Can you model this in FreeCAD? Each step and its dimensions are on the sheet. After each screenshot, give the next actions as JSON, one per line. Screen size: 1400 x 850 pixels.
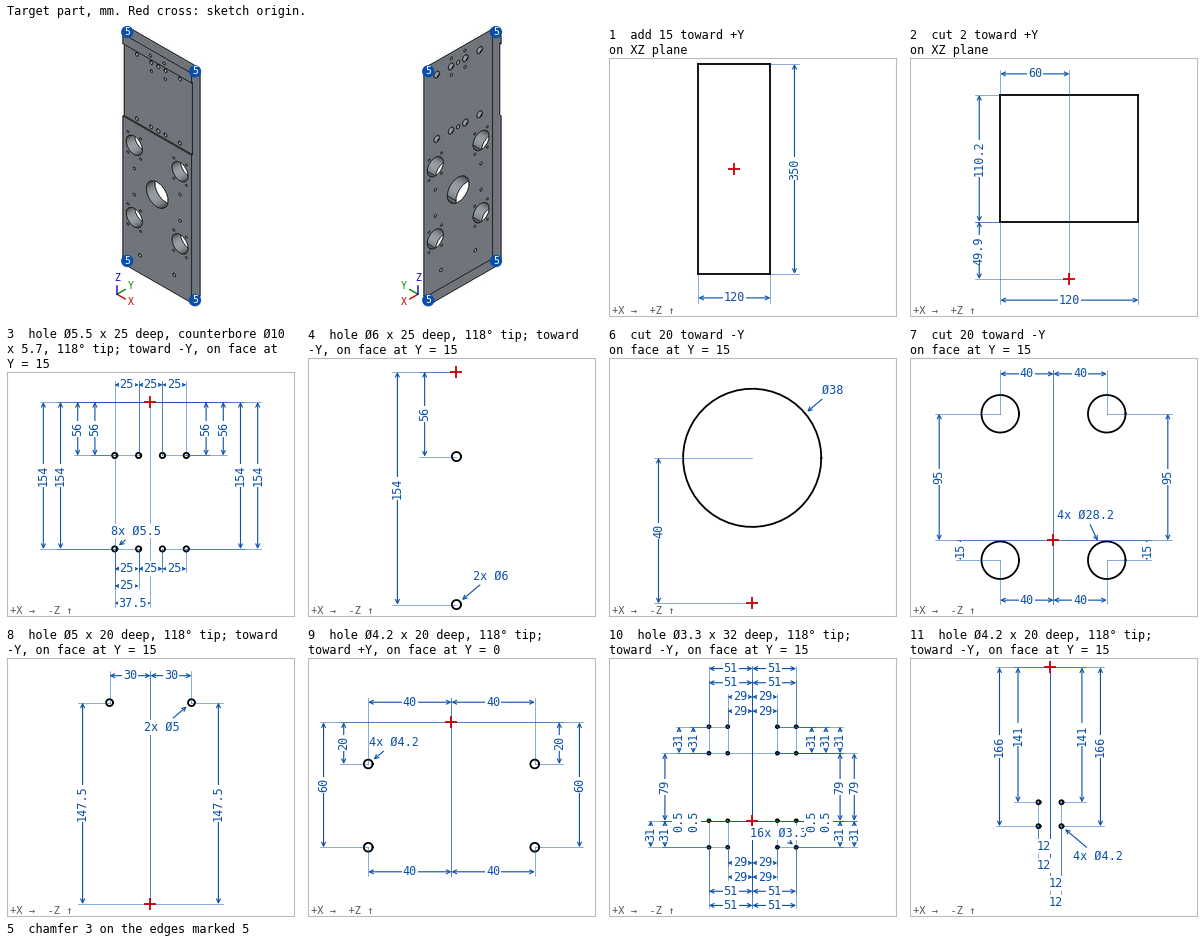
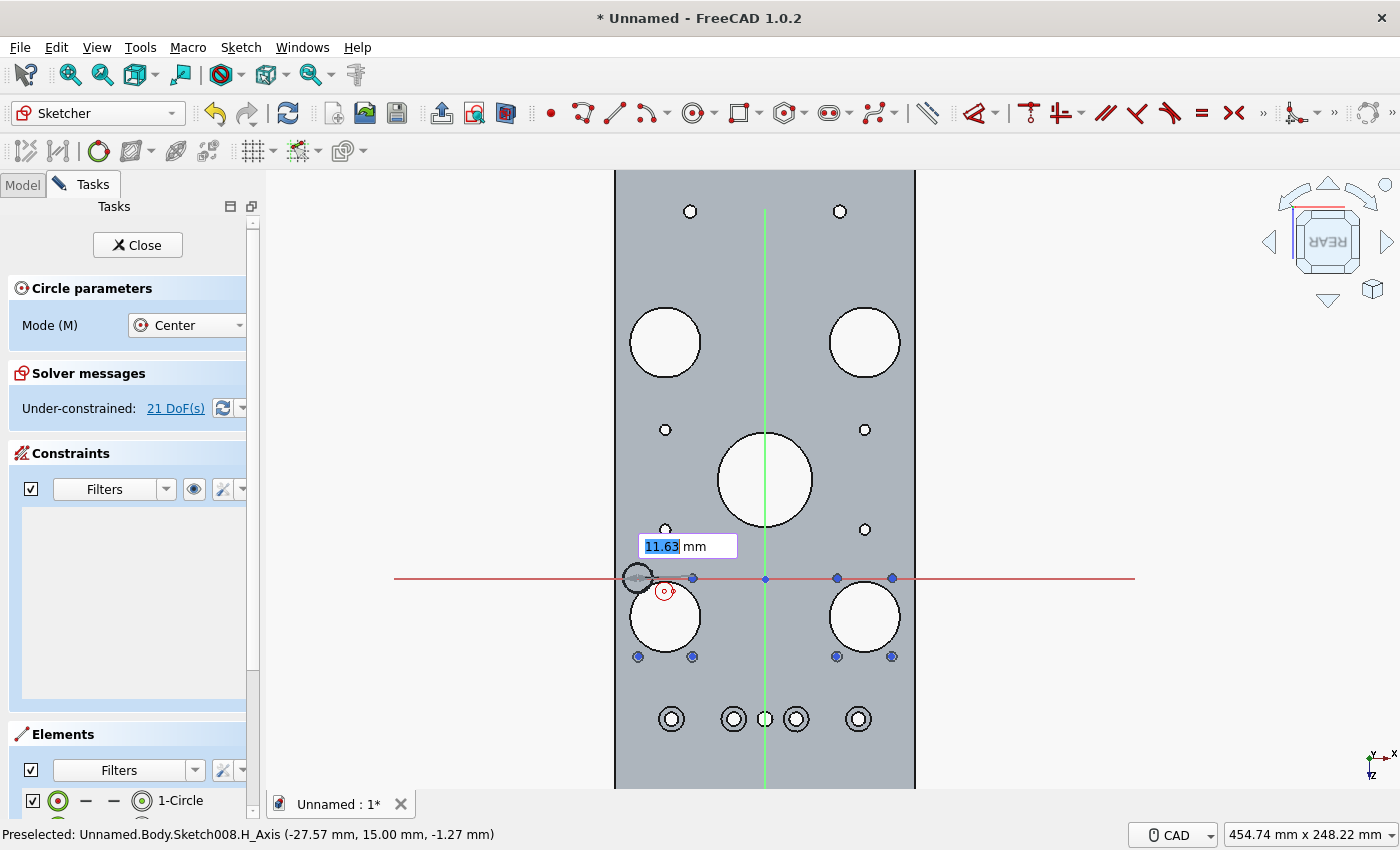
{"action": "scroll", "coordinate": [641, 575], "scroll_direction": "up", "scroll_amount": 7}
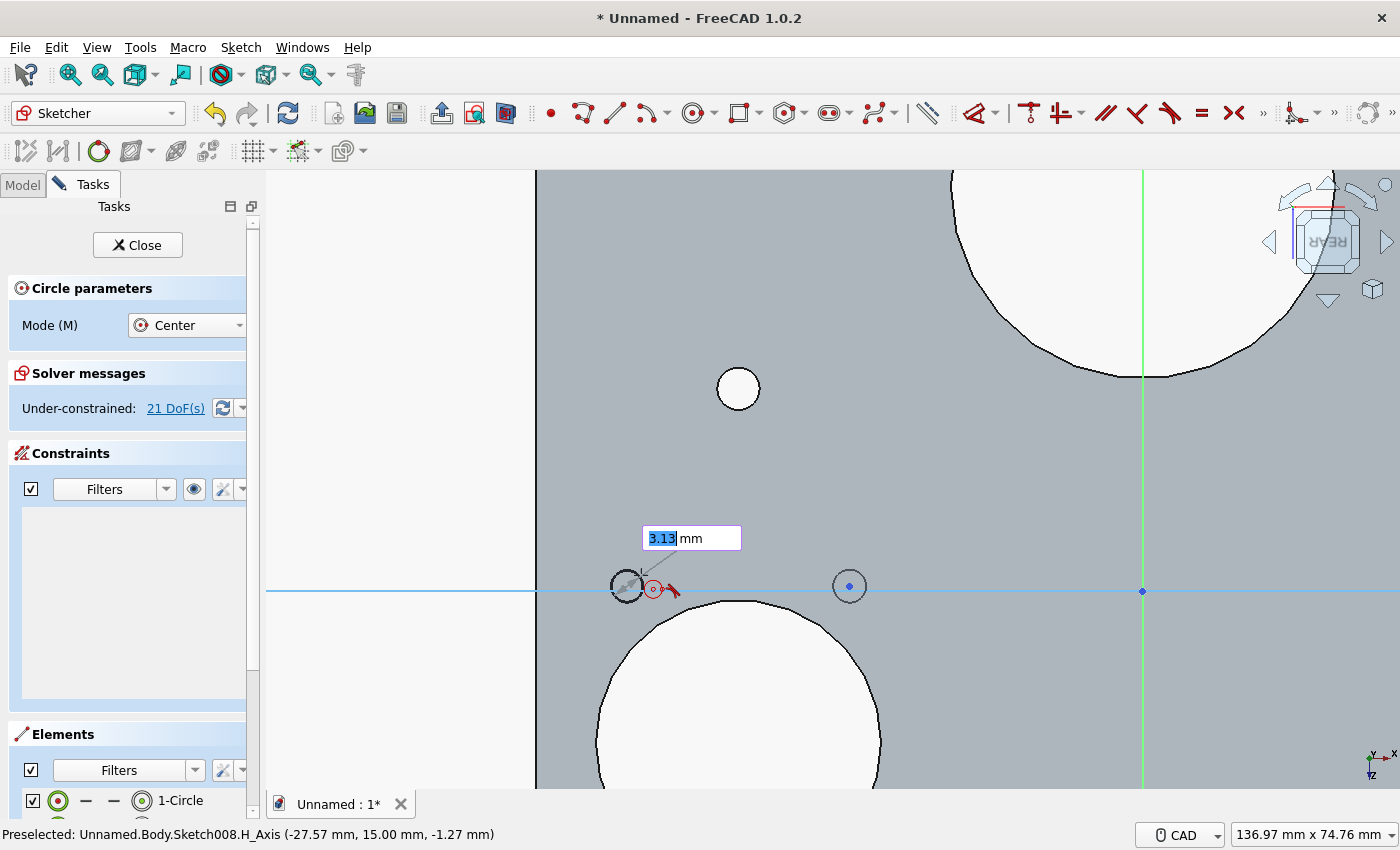
{"action": "left_click", "coordinate": [639, 574]}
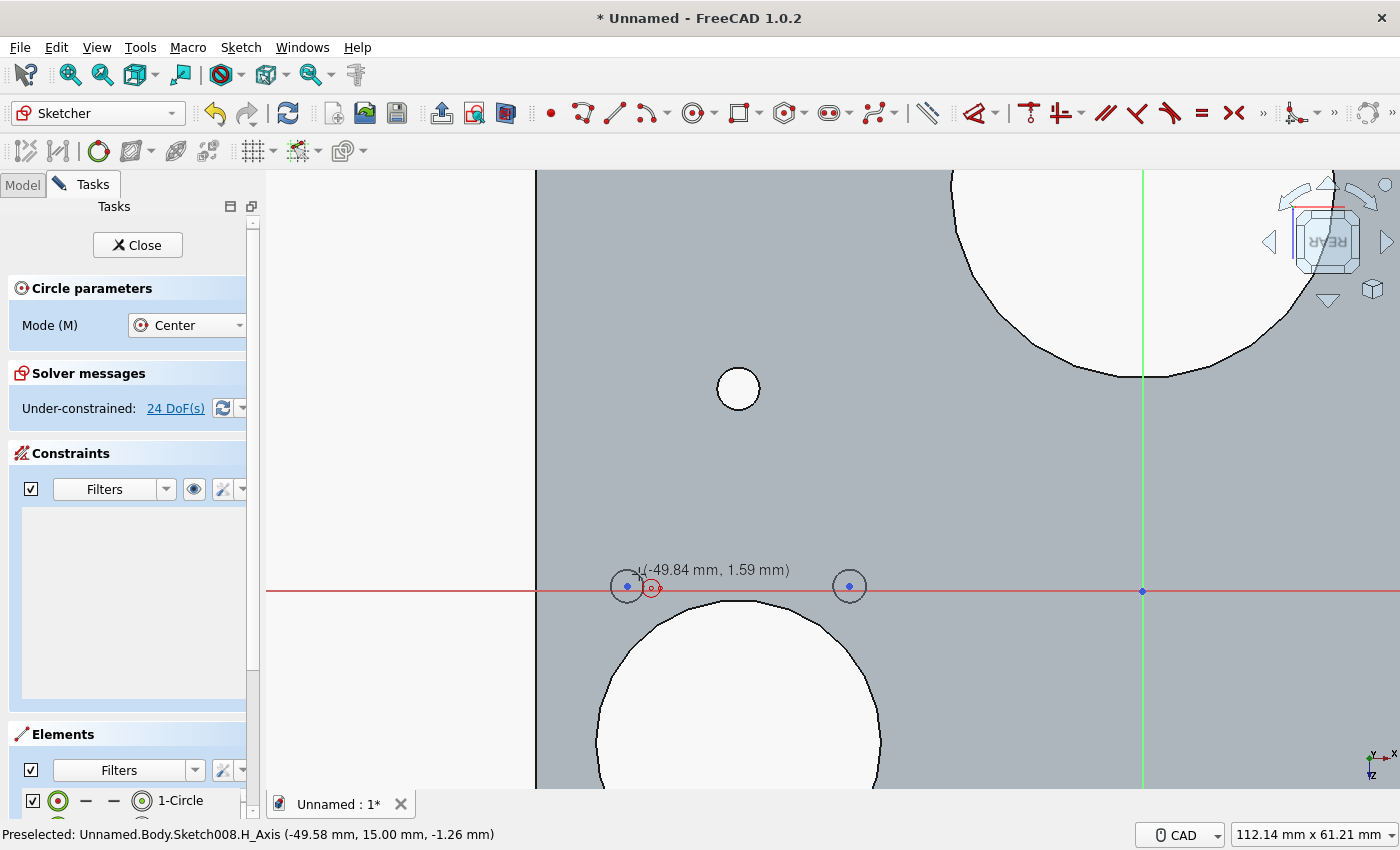
{"action": "scroll", "coordinate": [641, 575], "scroll_direction": "down", "scroll_amount": 7}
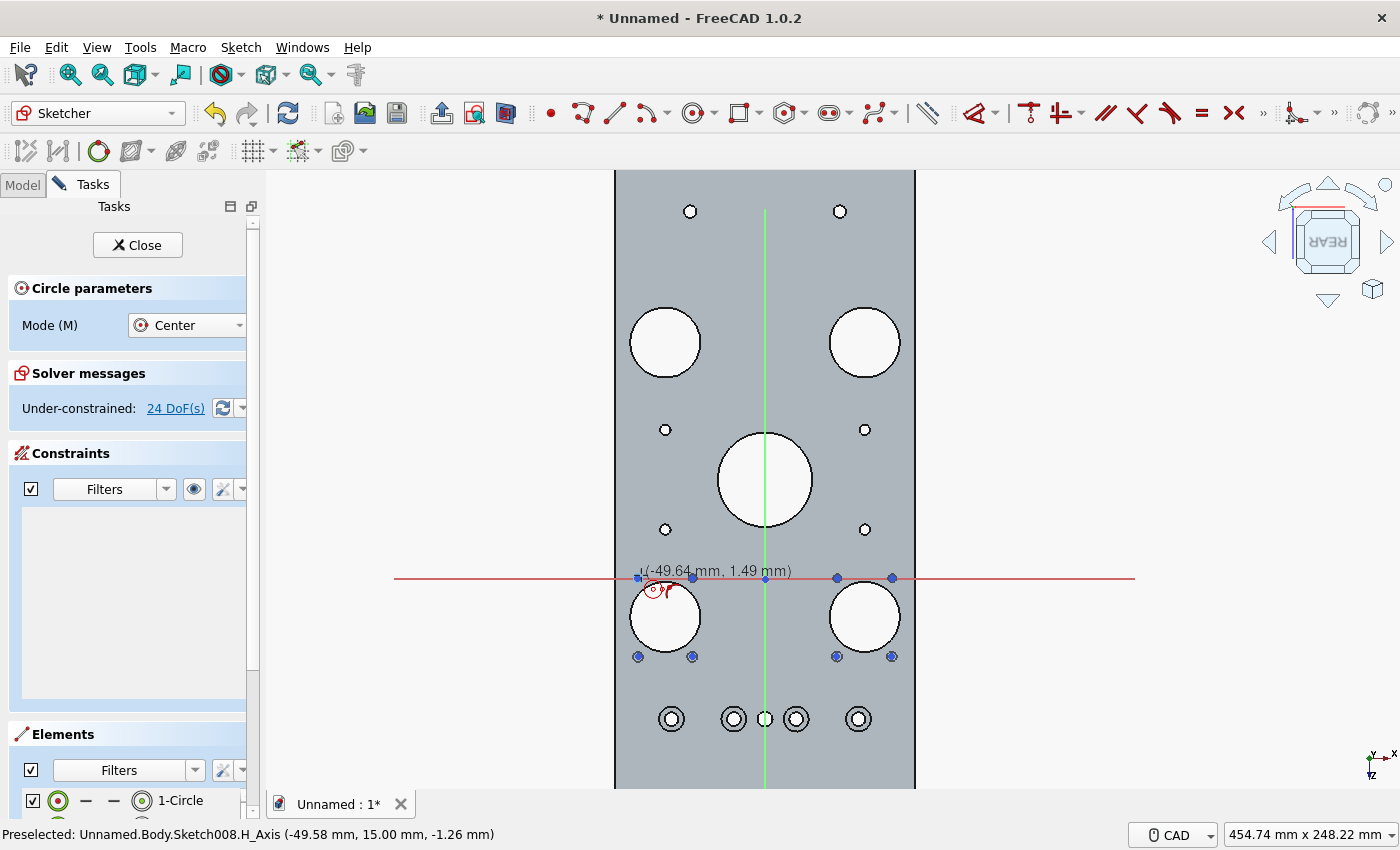
{"action": "scroll", "coordinate": [892, 381], "scroll_direction": "up", "scroll_amount": 9}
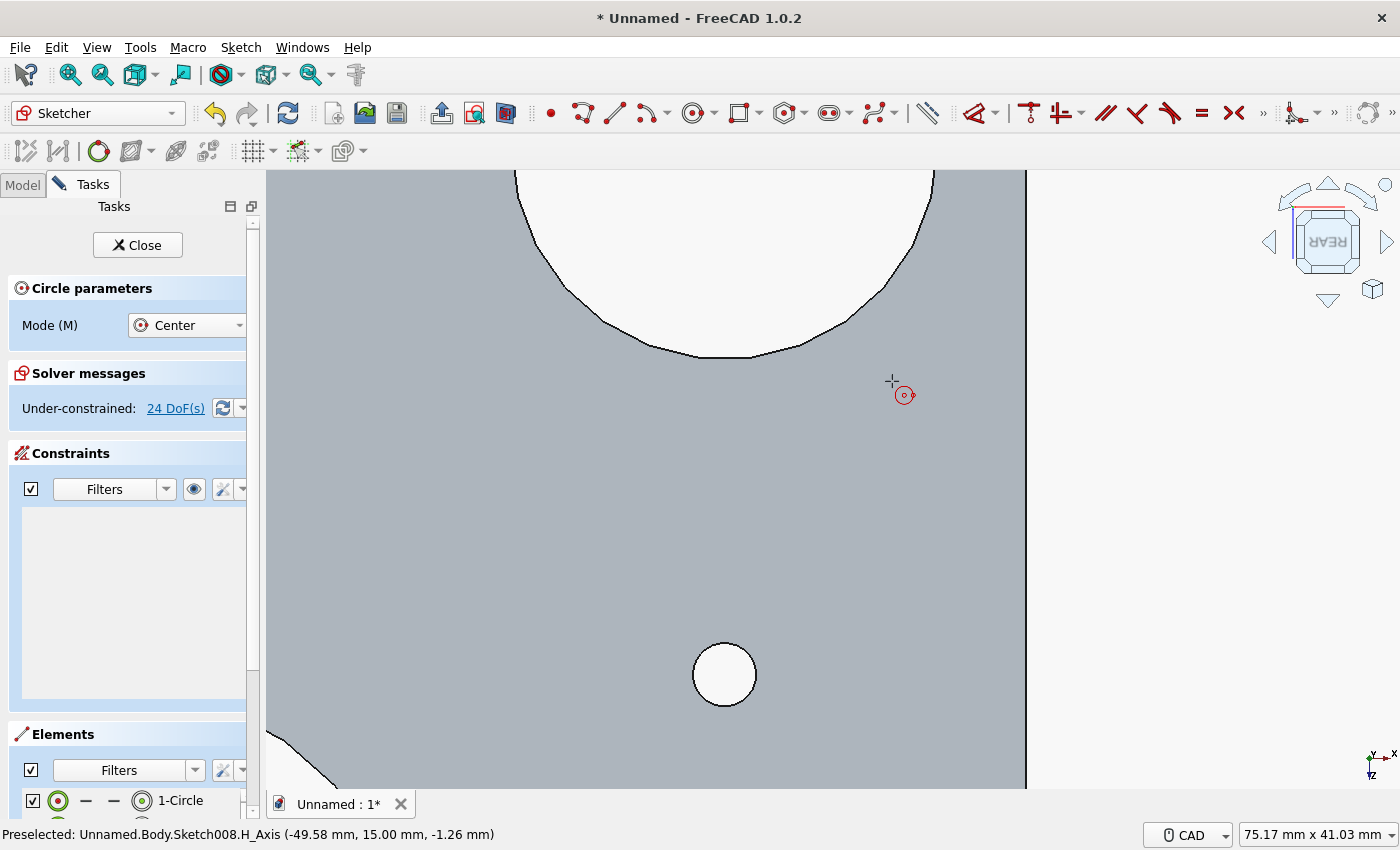
{"action": "scroll", "coordinate": [892, 381], "scroll_direction": "down", "scroll_amount": 9}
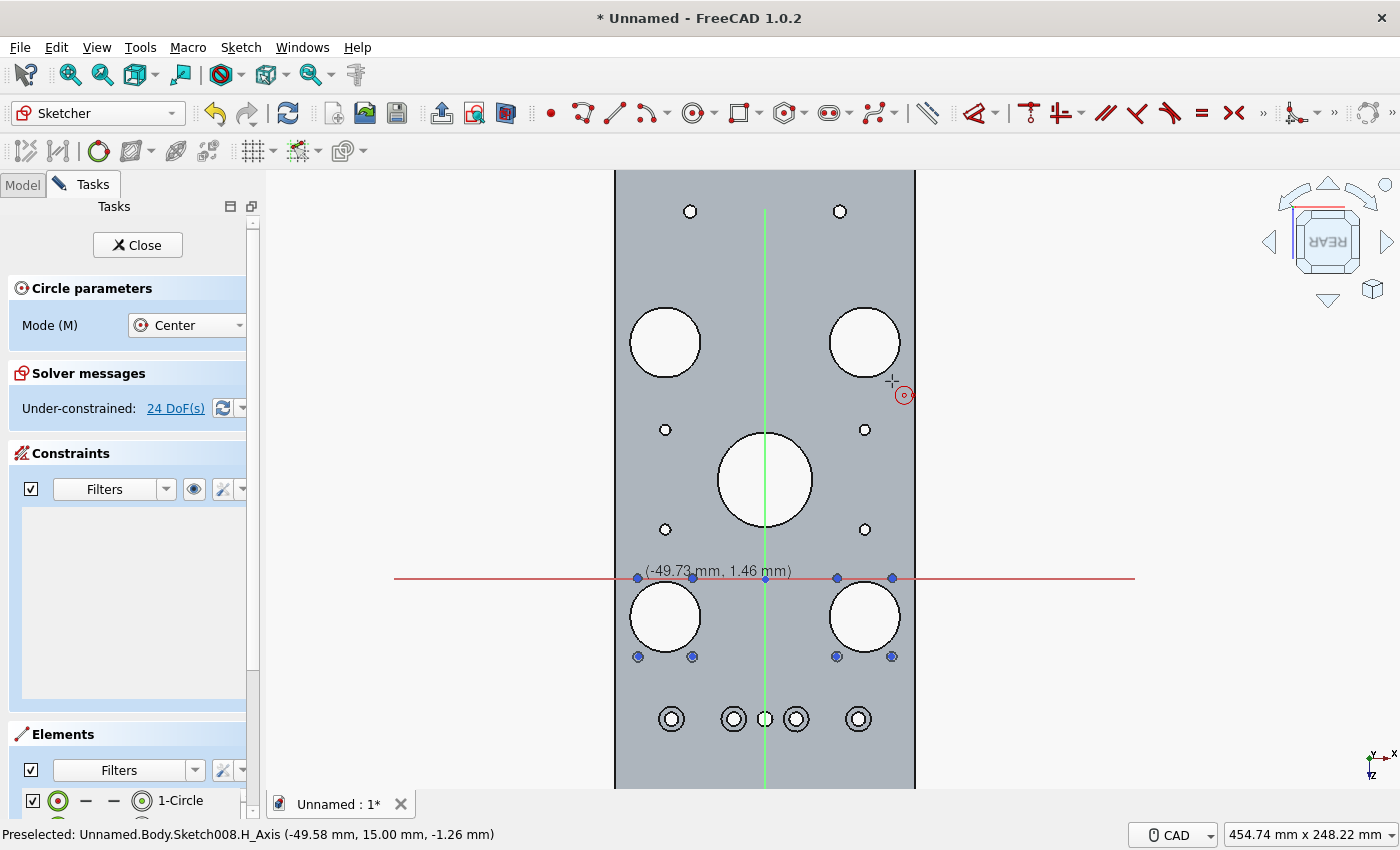
{"action": "left_click", "coordinate": [892, 381]}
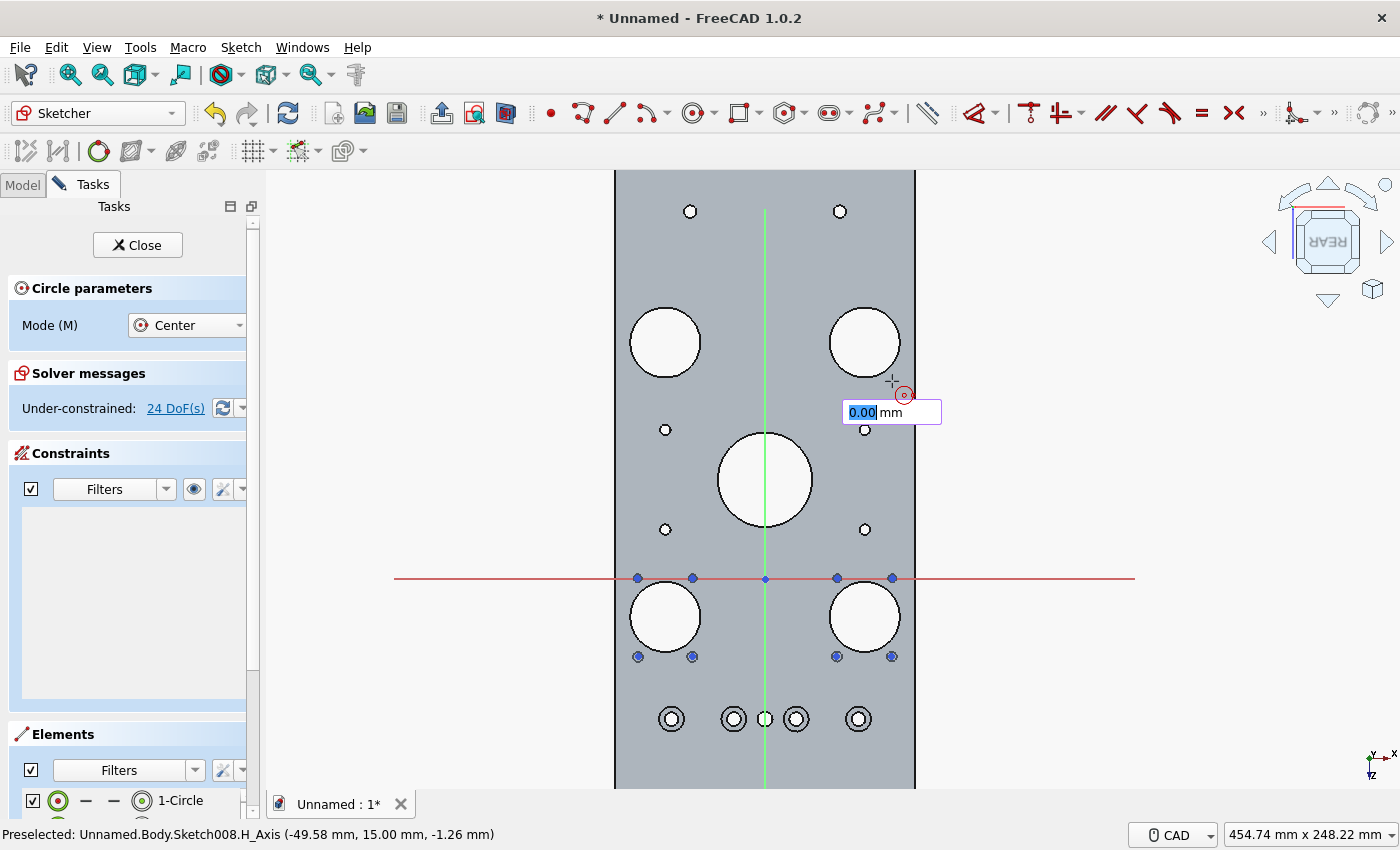
{"action": "scroll", "coordinate": [895, 378], "scroll_direction": "up", "scroll_amount": 7}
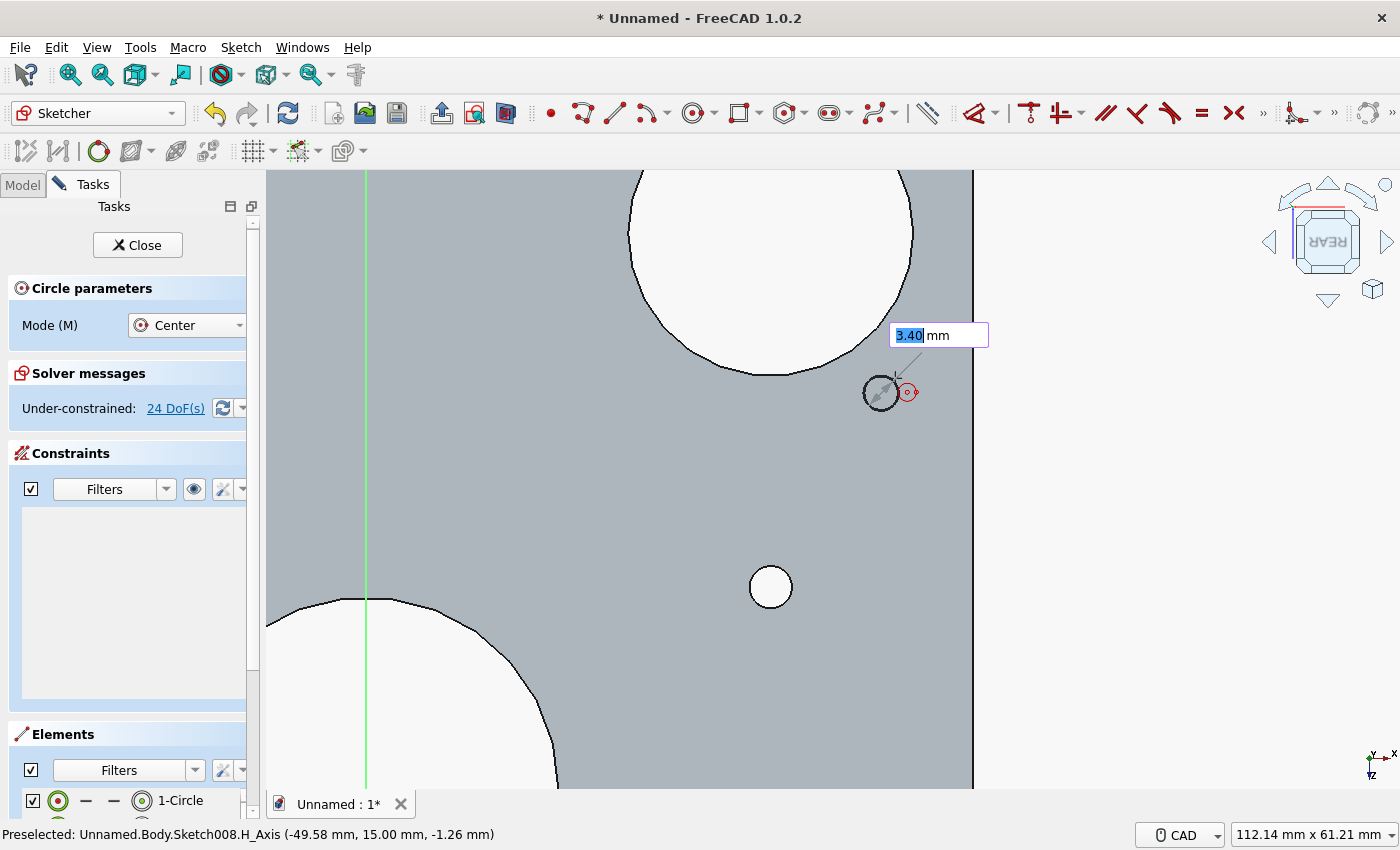
{"action": "left_click", "coordinate": [894, 378]}